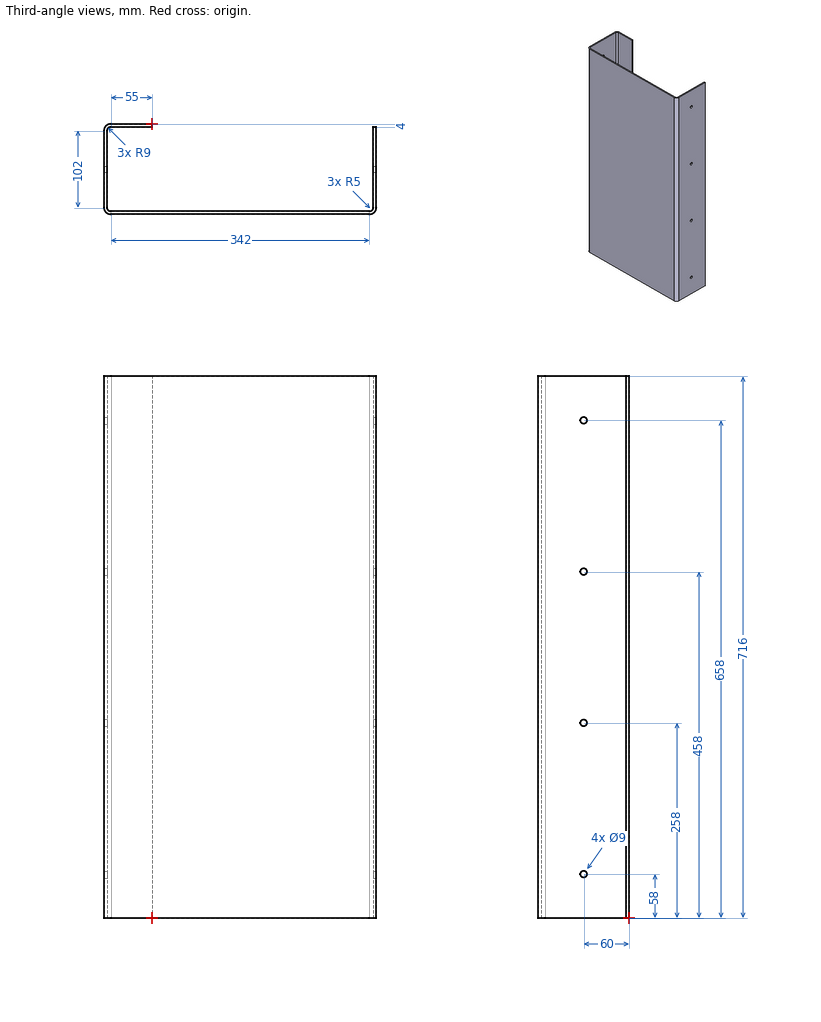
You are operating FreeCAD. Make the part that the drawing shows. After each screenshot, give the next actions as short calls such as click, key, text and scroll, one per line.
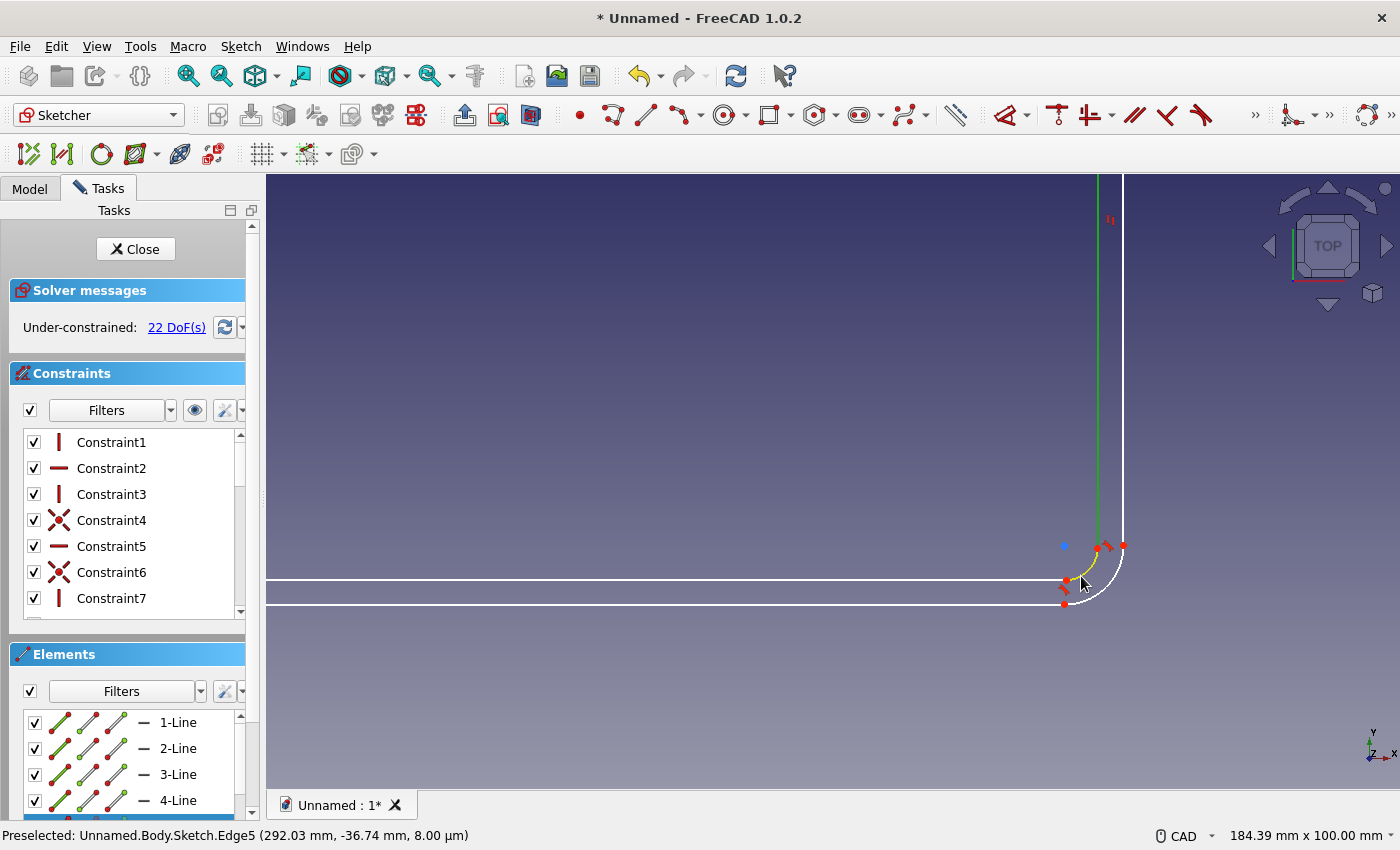
click(1081, 576)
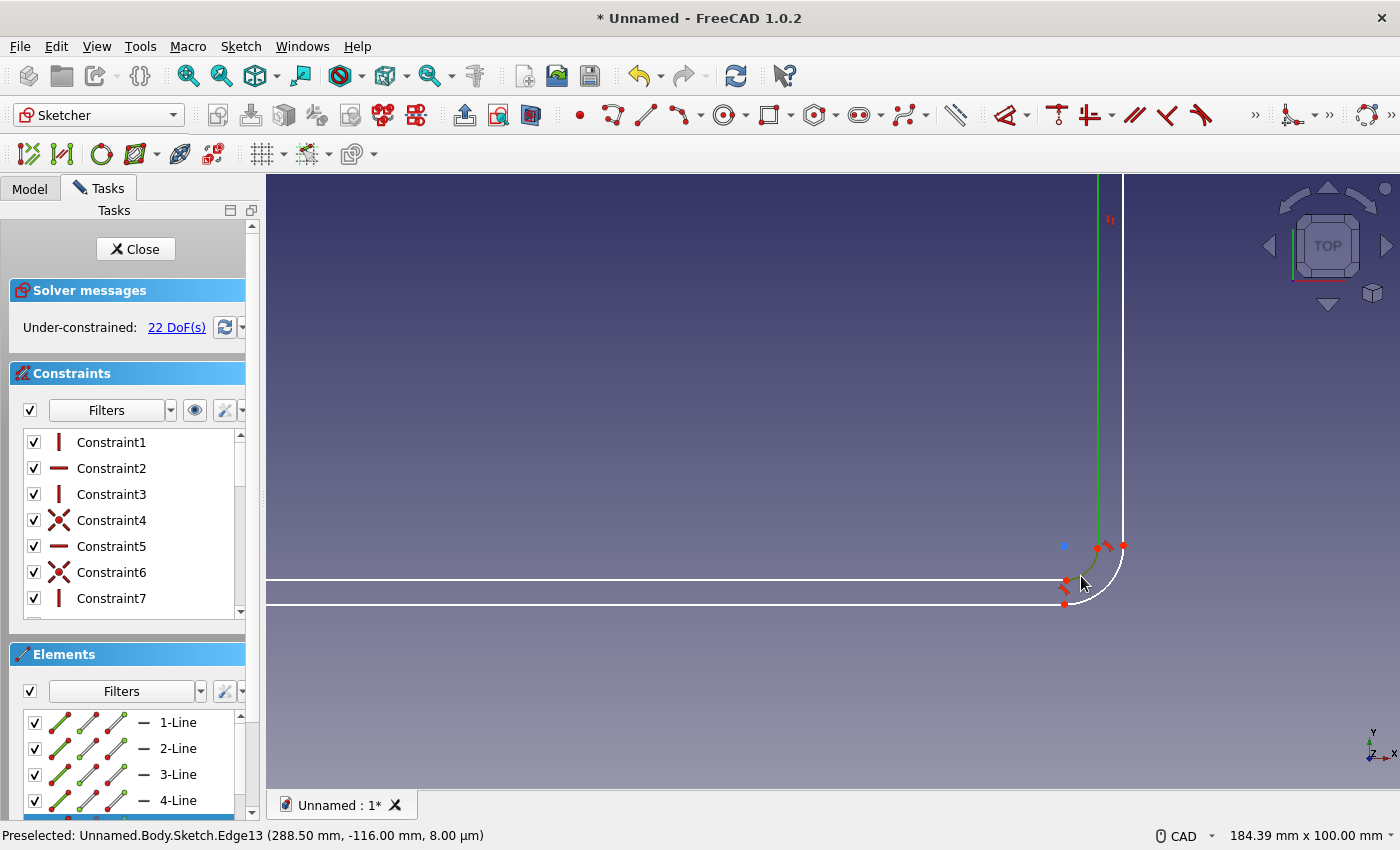
click(1201, 116)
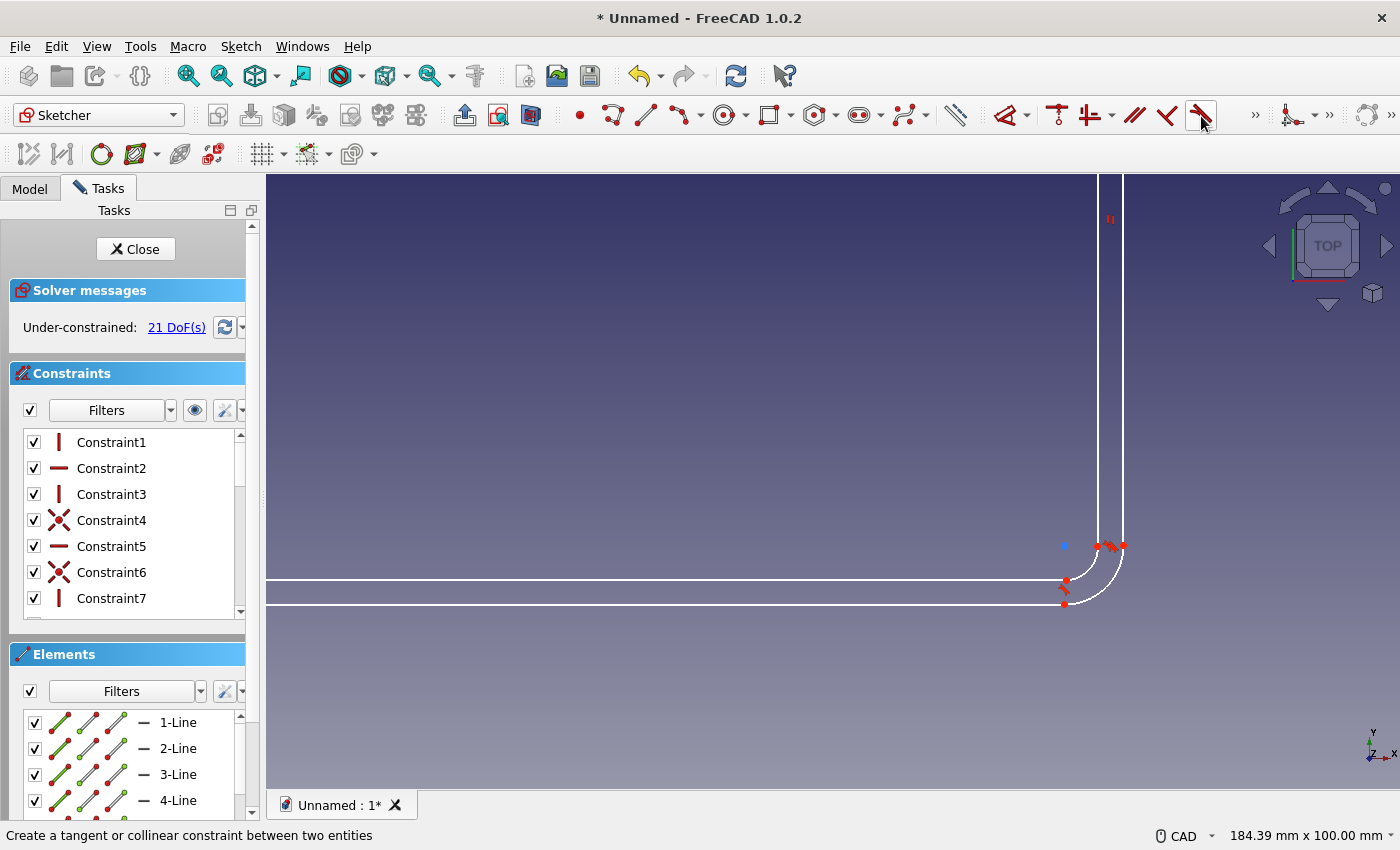
click(436, 580)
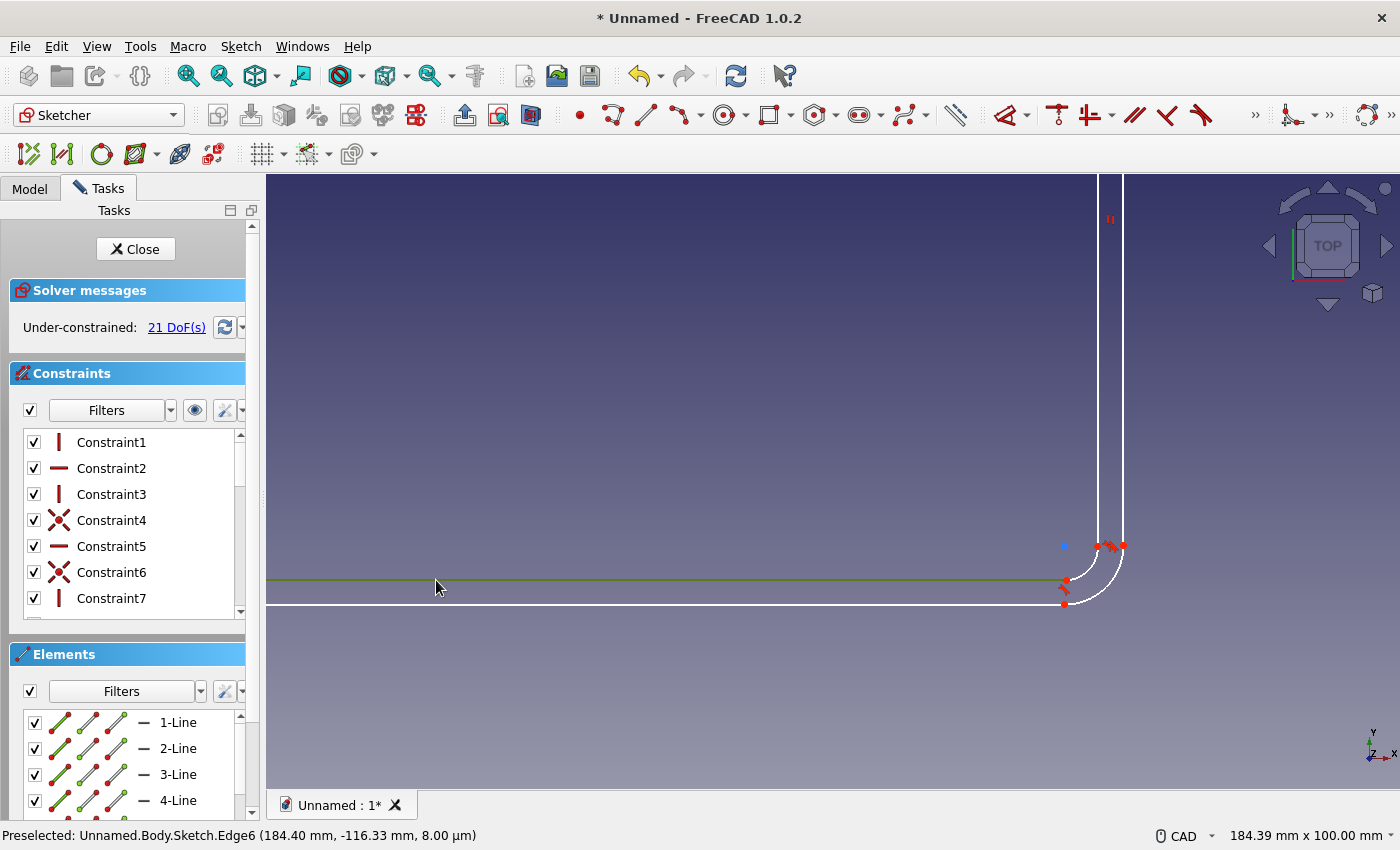
click(1081, 576)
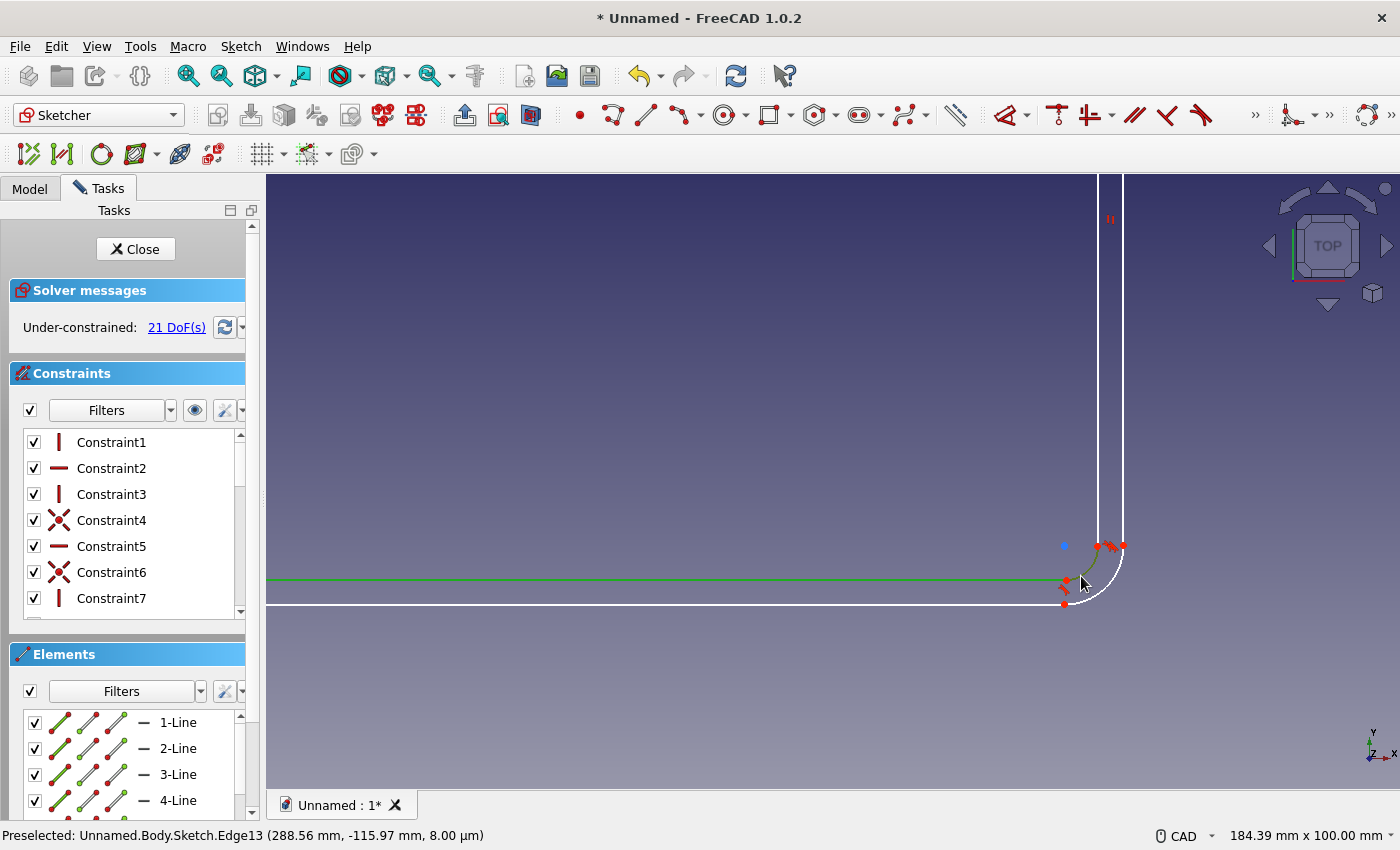
click(1201, 116)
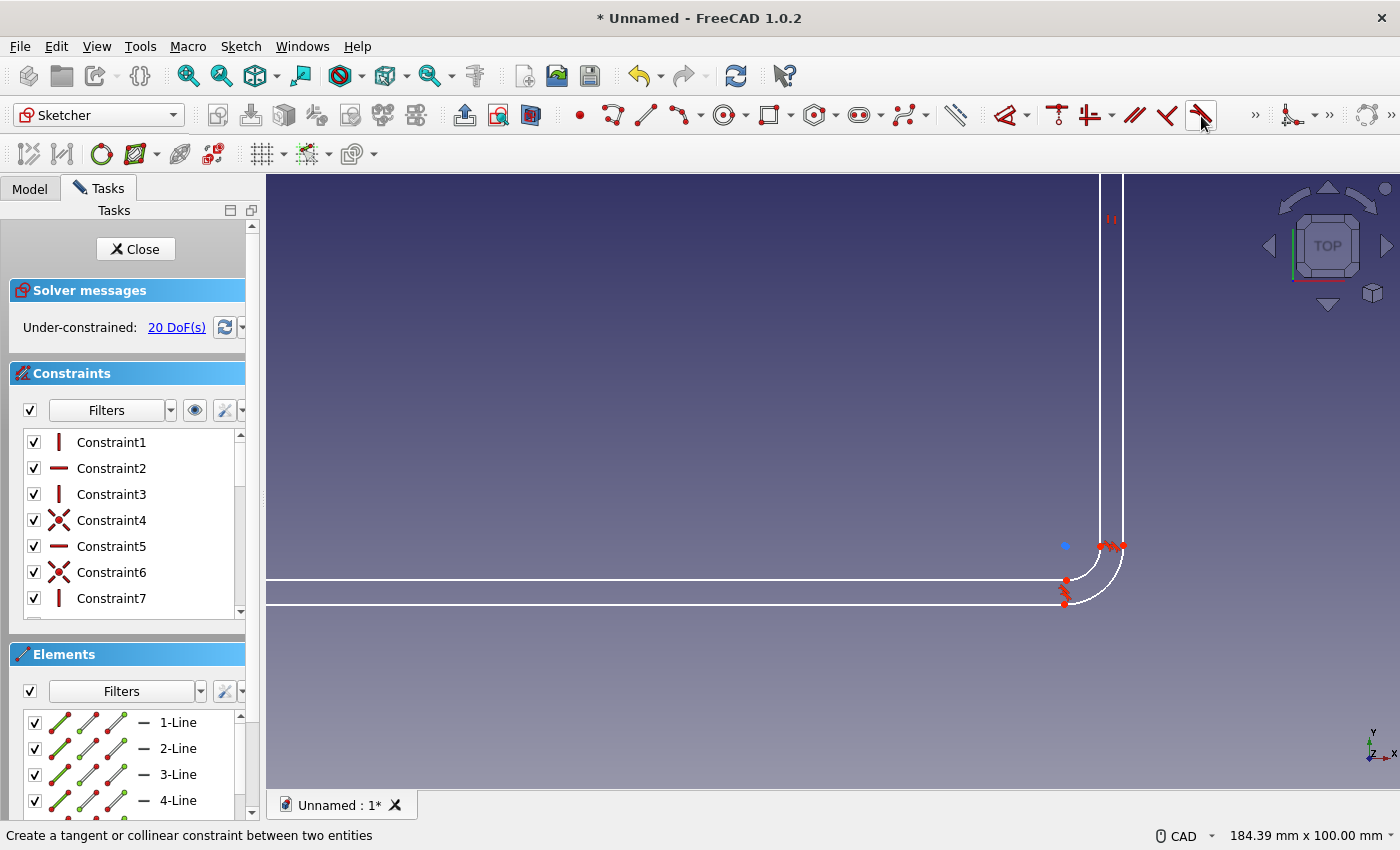
click(436, 580)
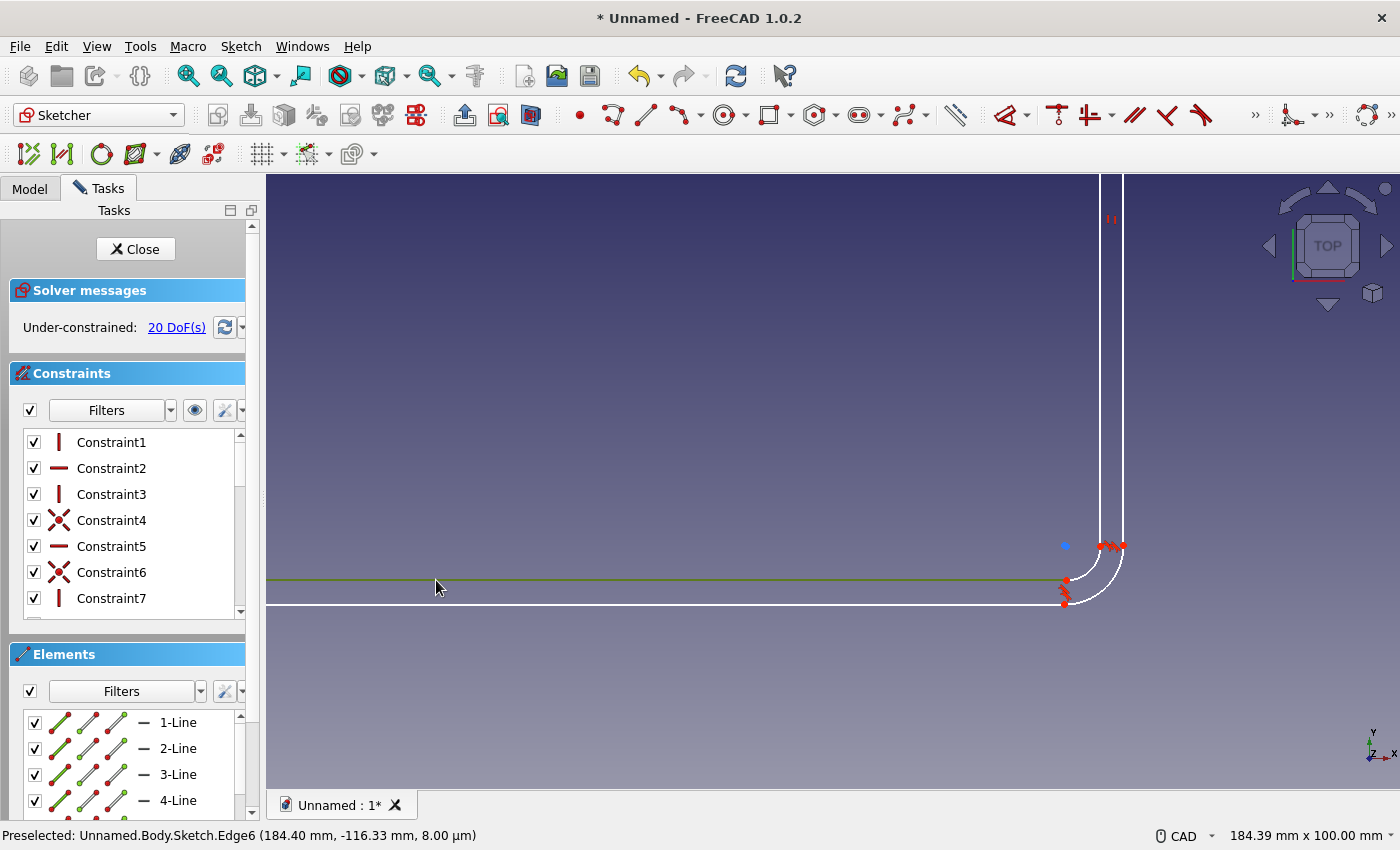
scroll(1087, 588, down, 6)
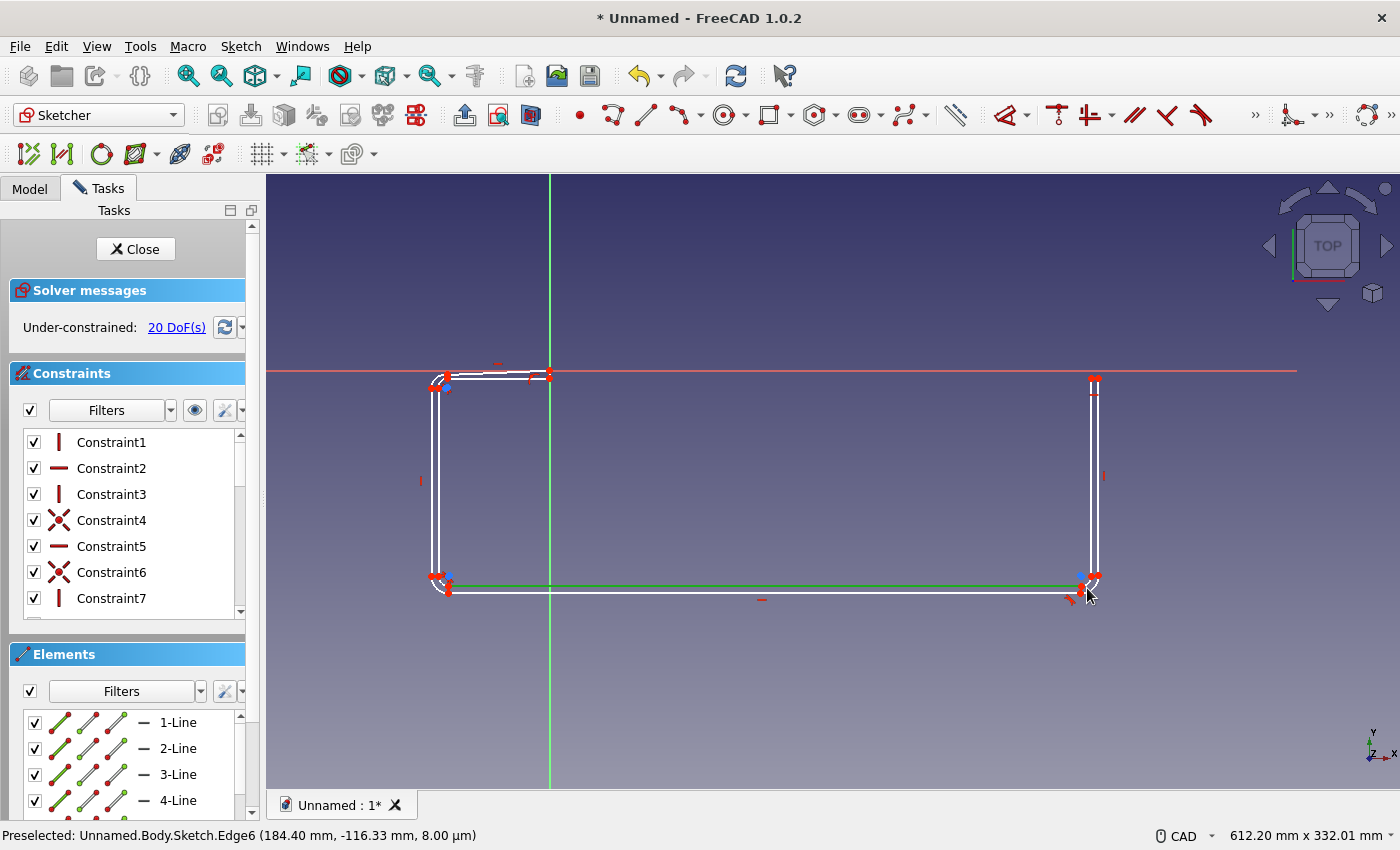
scroll(440, 581, up, 6)